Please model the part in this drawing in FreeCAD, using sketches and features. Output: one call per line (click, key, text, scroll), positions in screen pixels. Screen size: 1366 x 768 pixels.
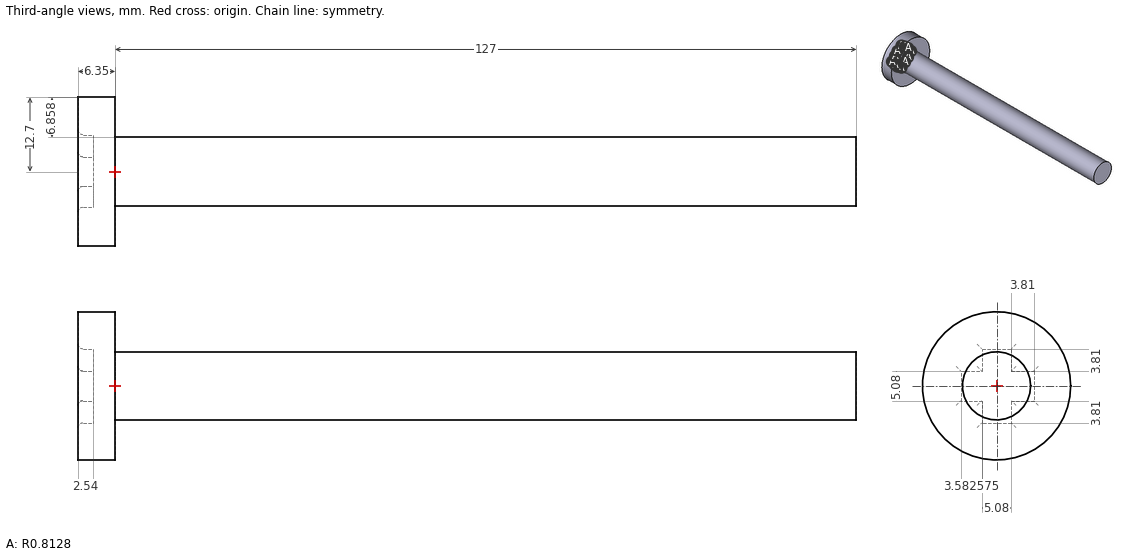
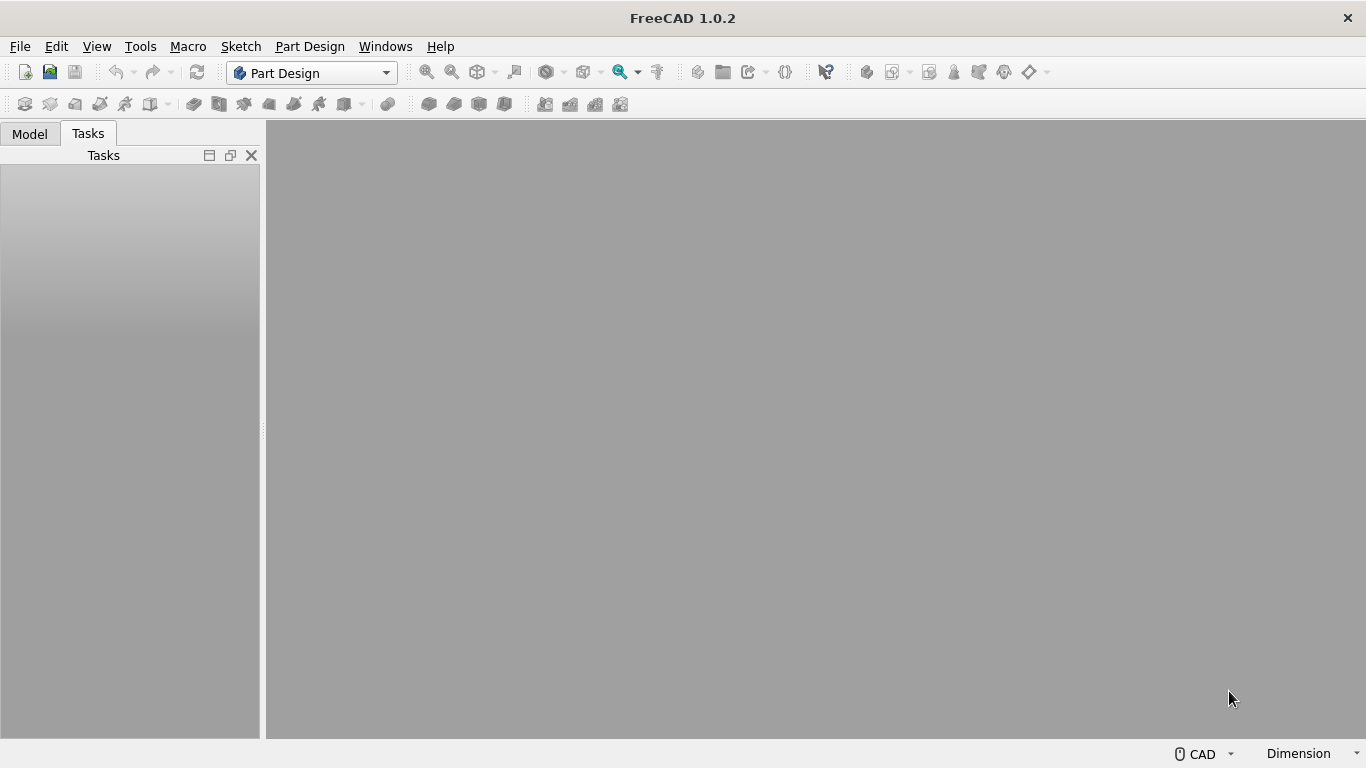
click(25, 72)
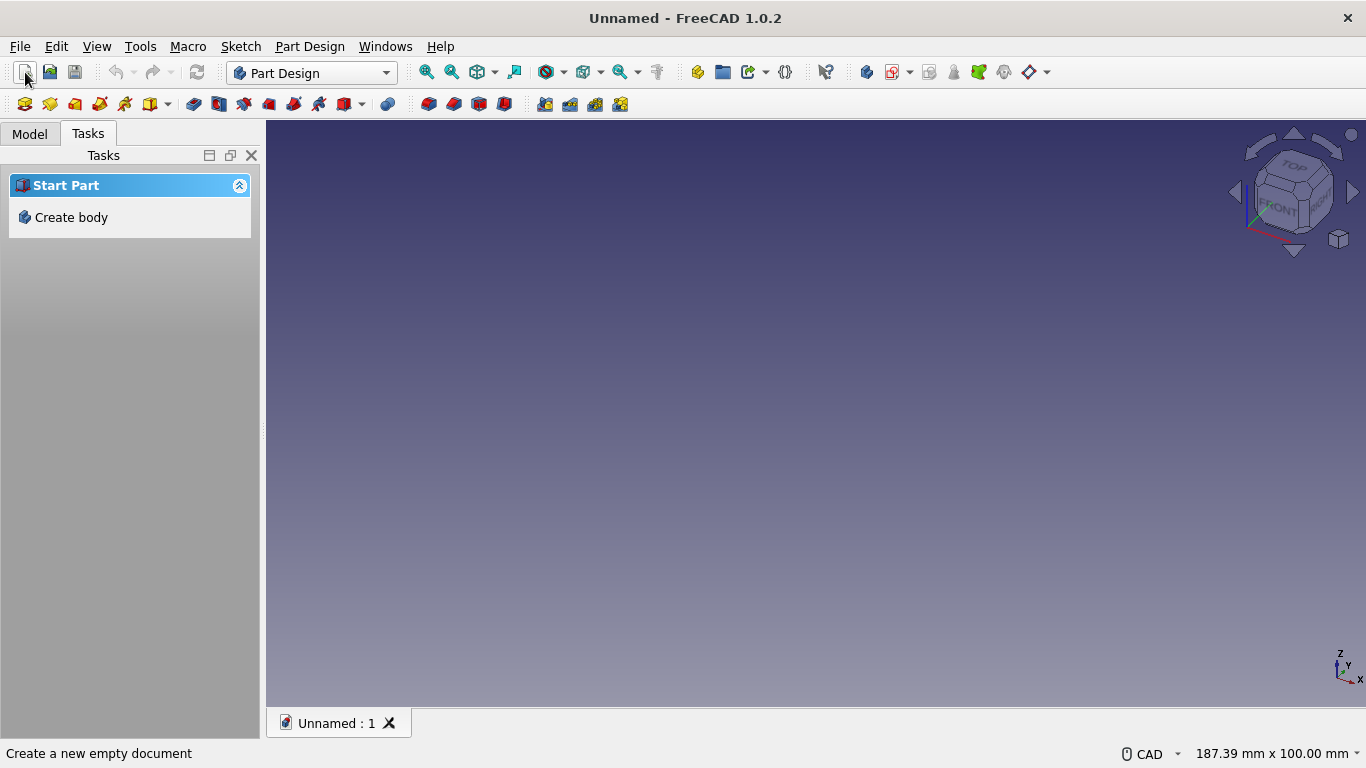
click(892, 72)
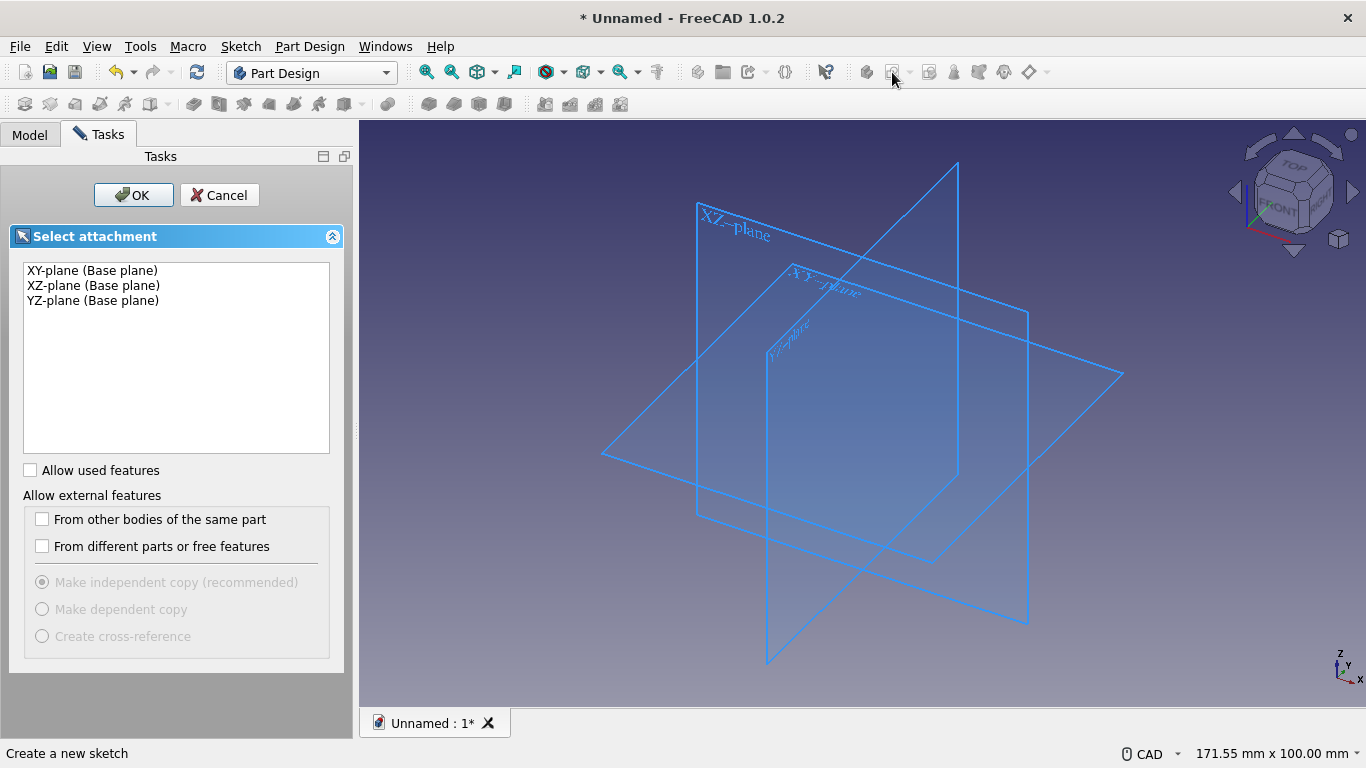
click(84, 270)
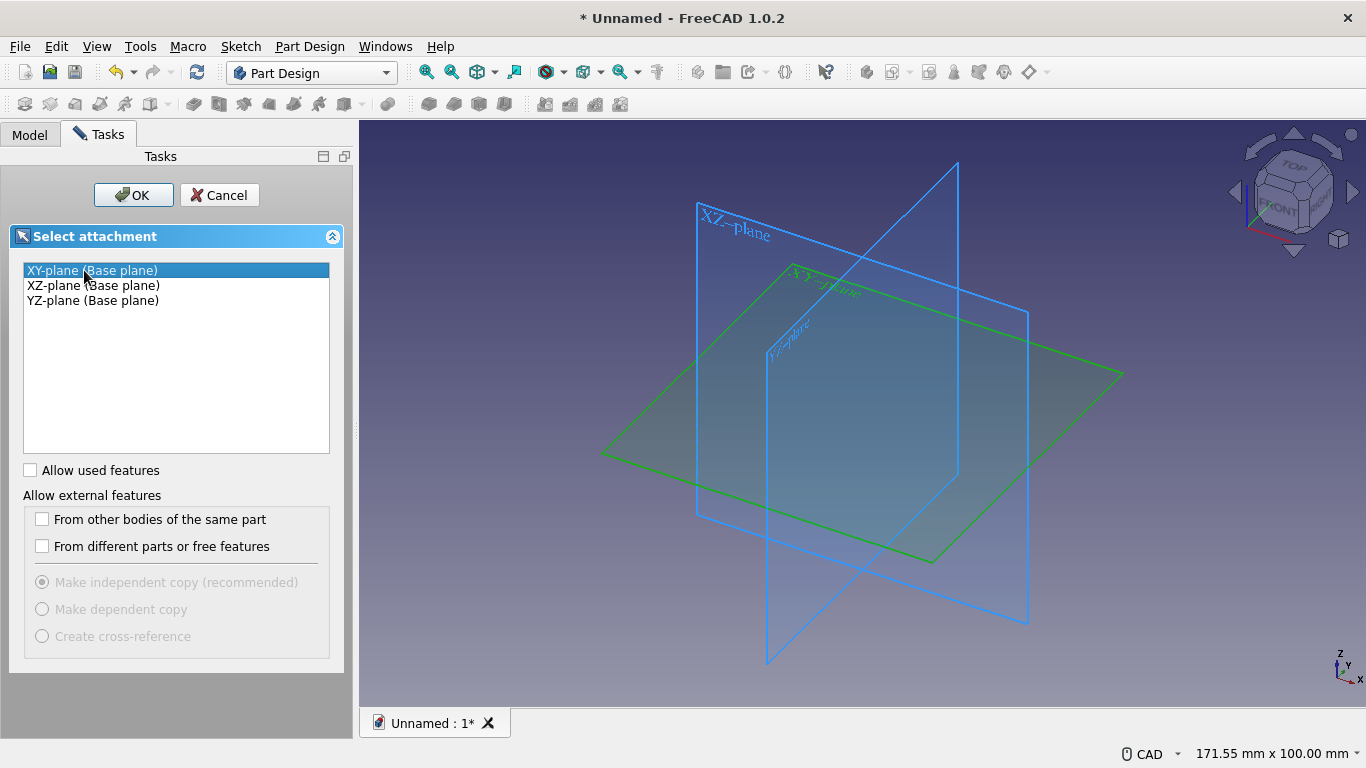
click(134, 195)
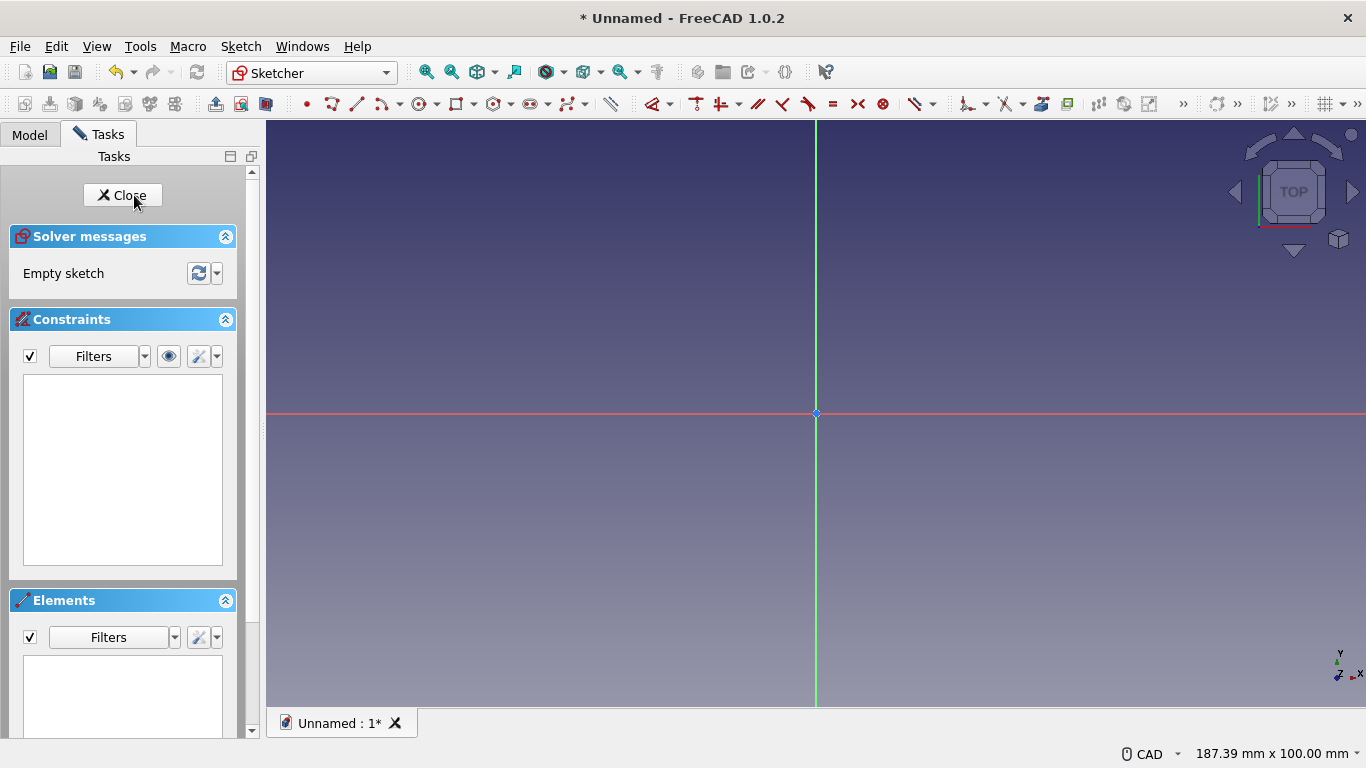
scroll(294, 489, down, 2)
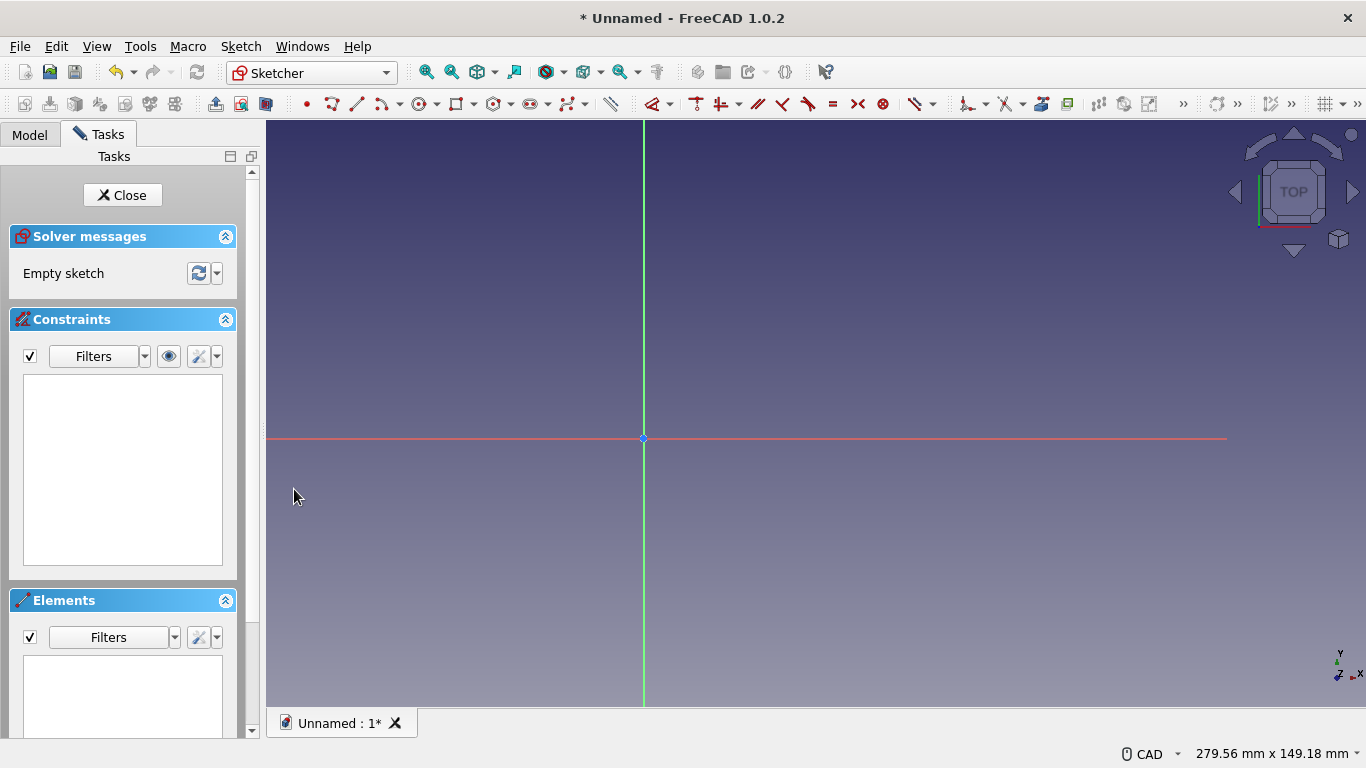
click(332, 104)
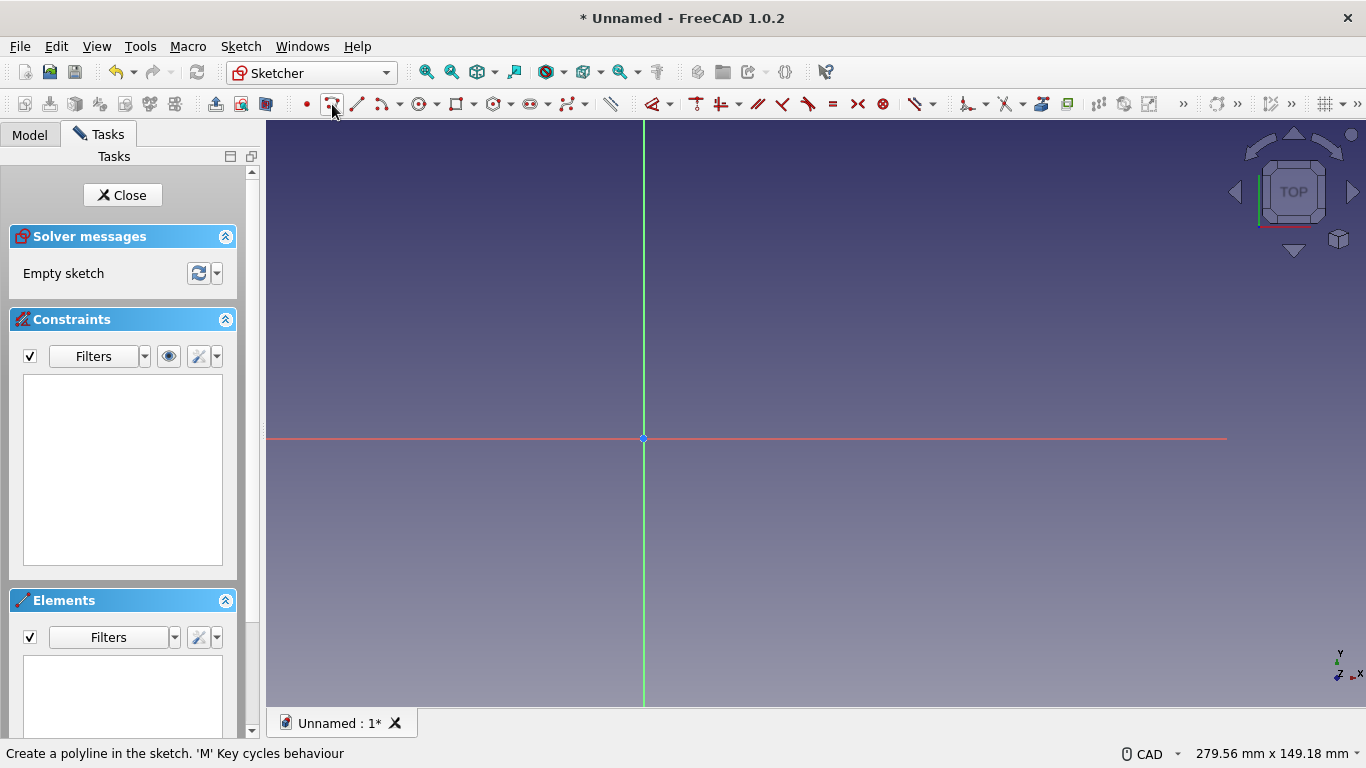
click(644, 416)
click(653, 389)
click(619, 389)
click(619, 439)
click(1144, 430)
click(1144, 416)
click(644, 417)
key(Escape)
key(Escape)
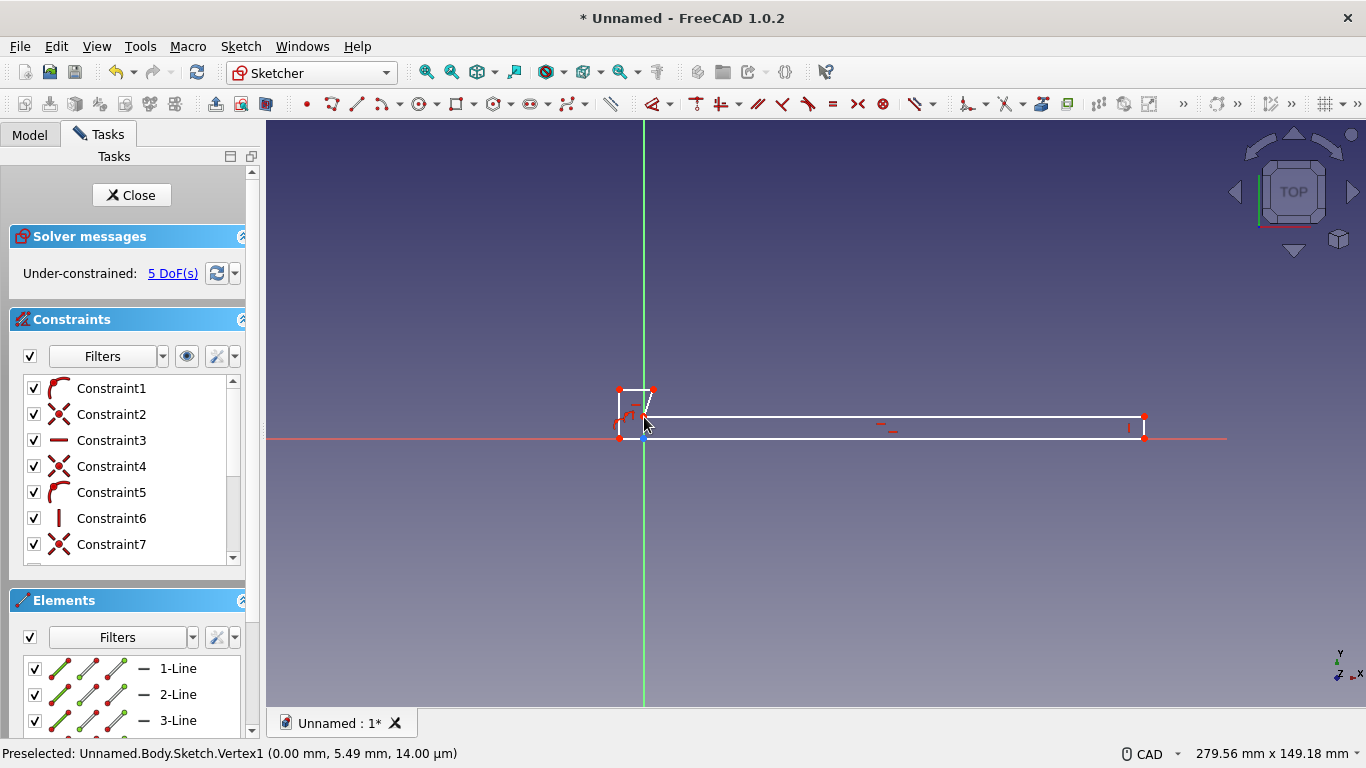
scroll(648, 406, up, 2)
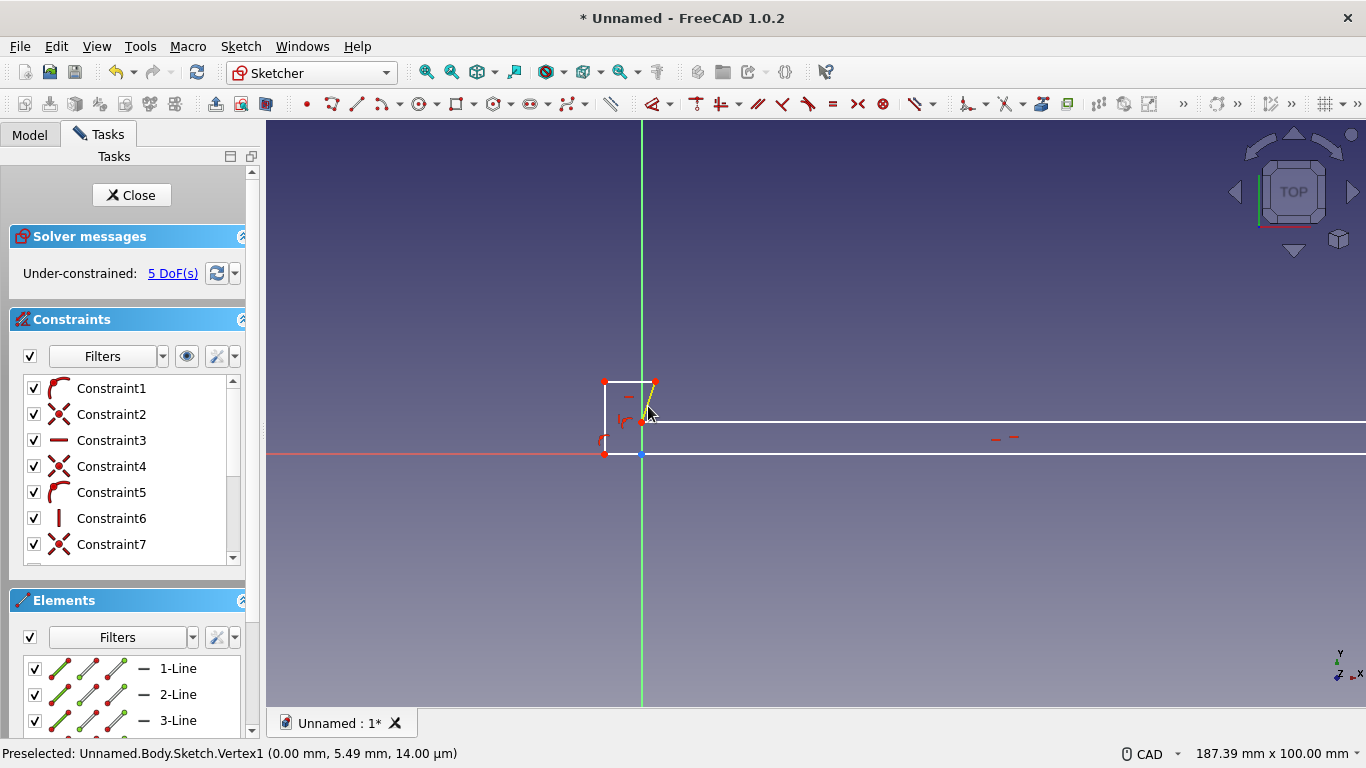
click(647, 406)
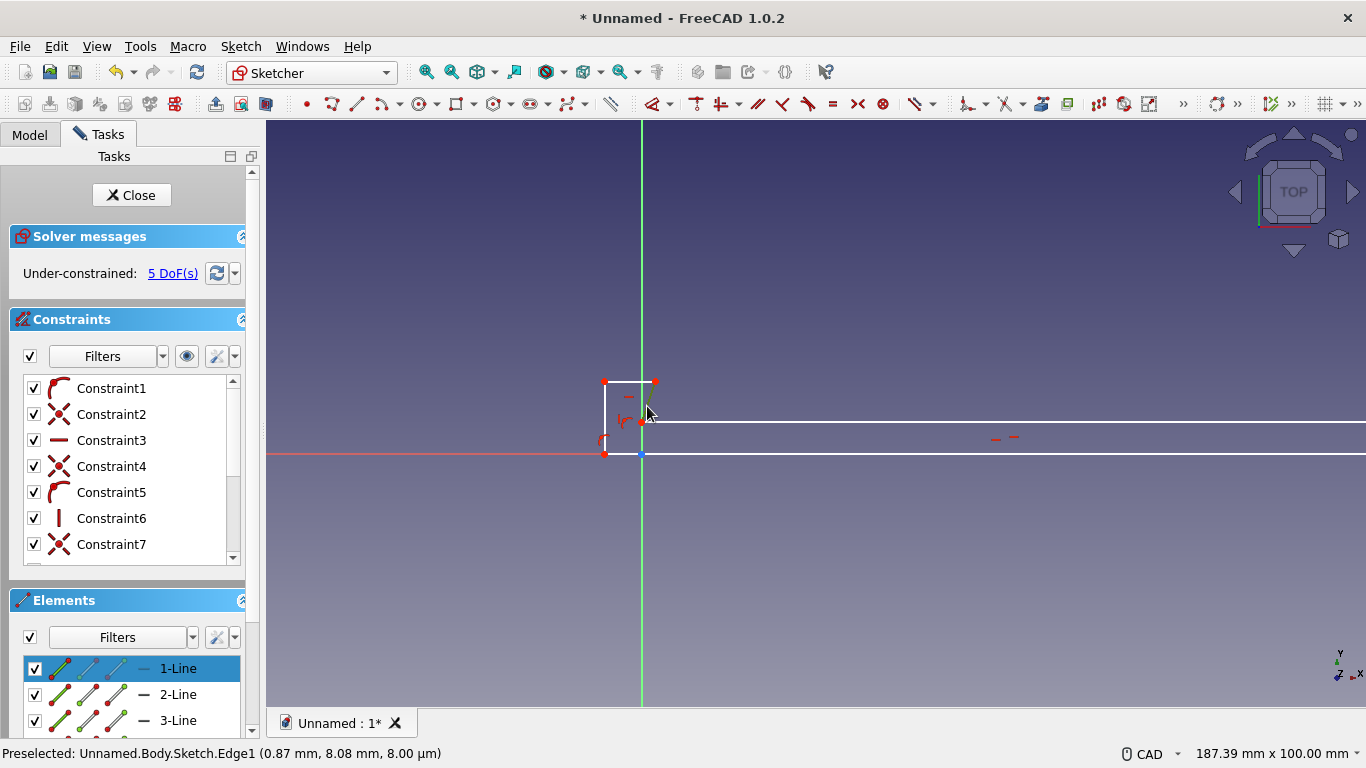
click(738, 104)